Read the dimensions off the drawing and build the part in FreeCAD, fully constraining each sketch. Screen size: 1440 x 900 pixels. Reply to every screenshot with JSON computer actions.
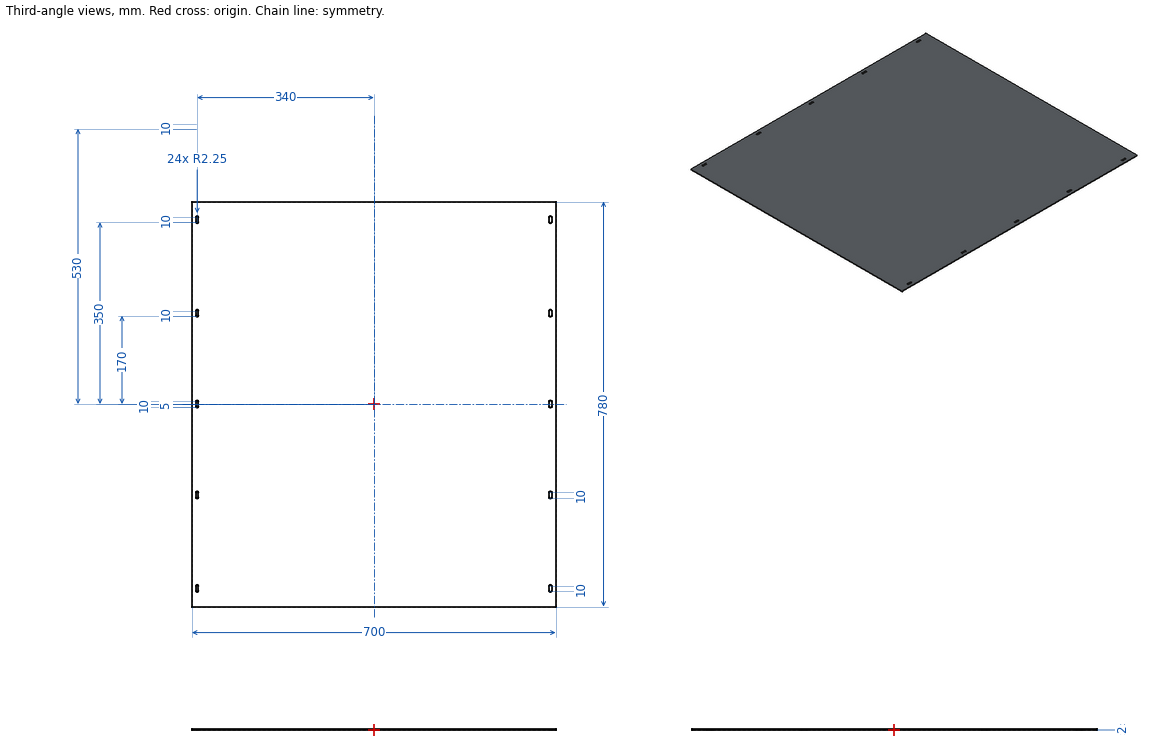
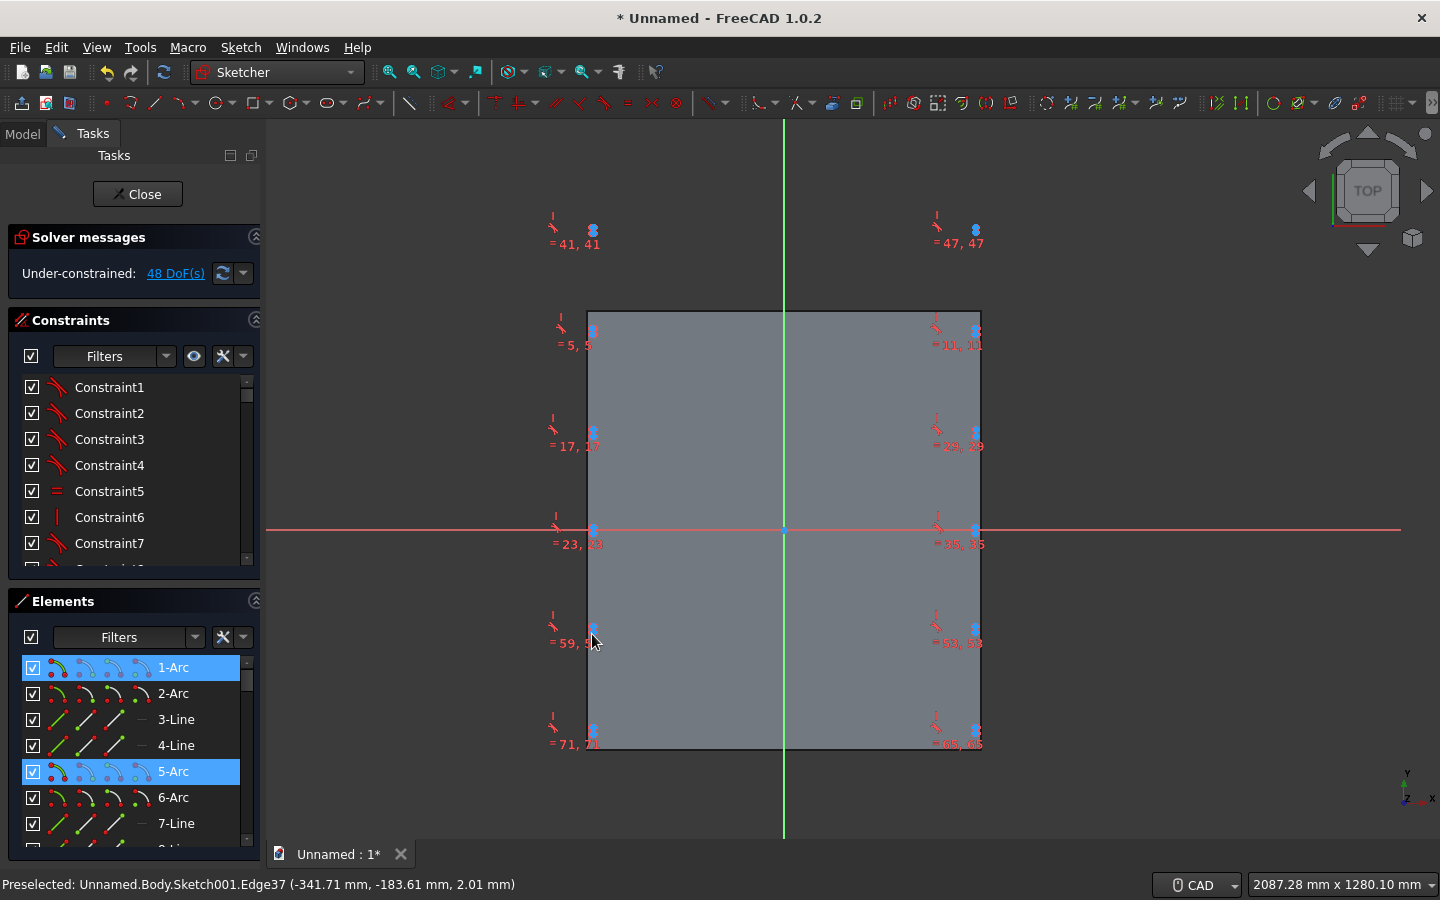
{"action": "scroll", "coordinate": [975, 735], "scroll_direction": "up", "scroll_amount": 12}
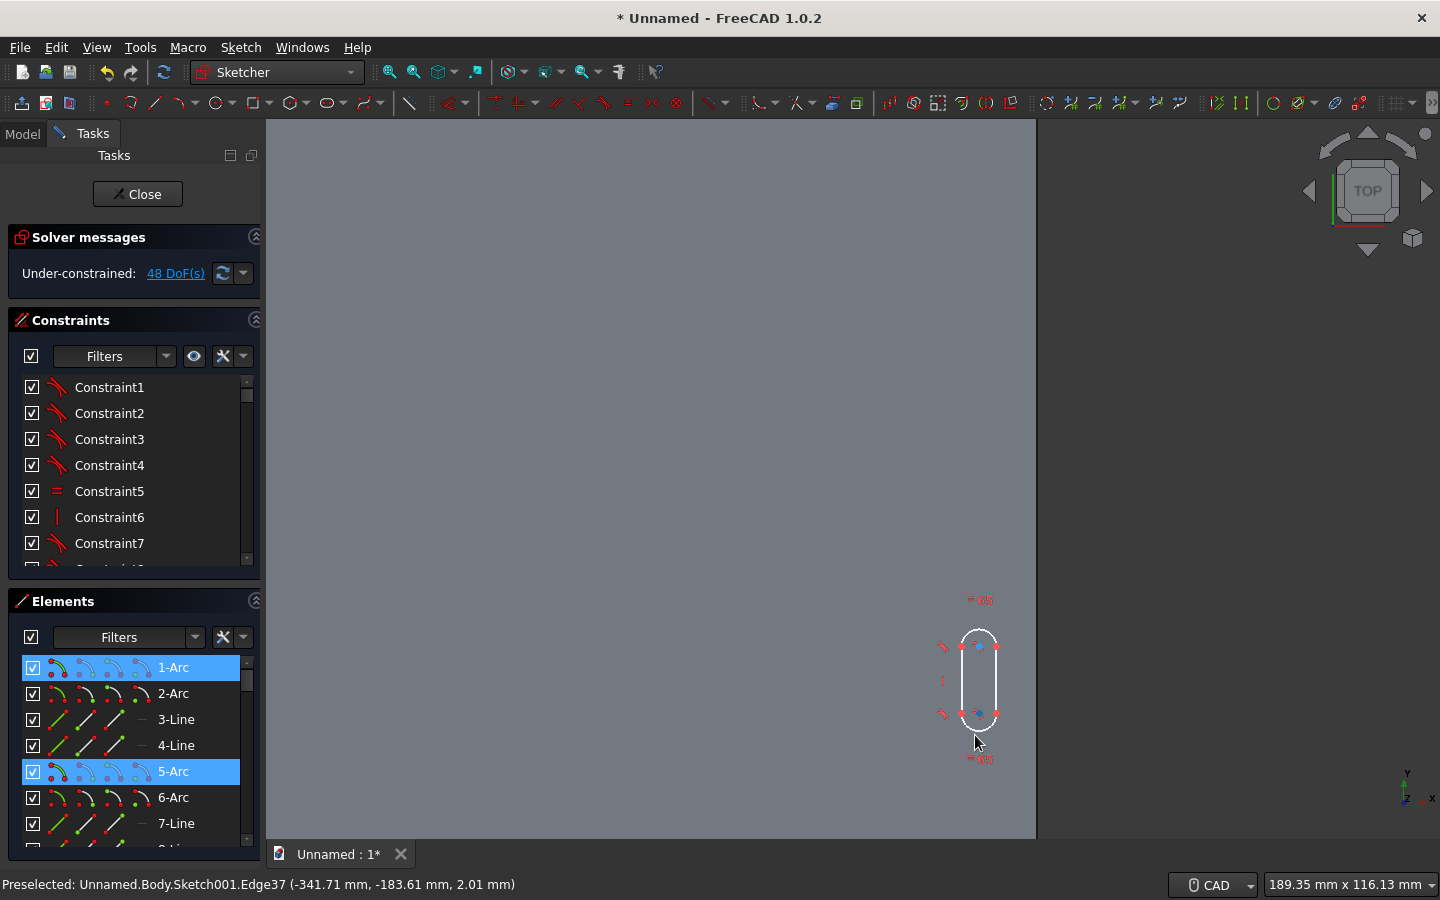
{"action": "left_click", "coordinate": [969, 728]}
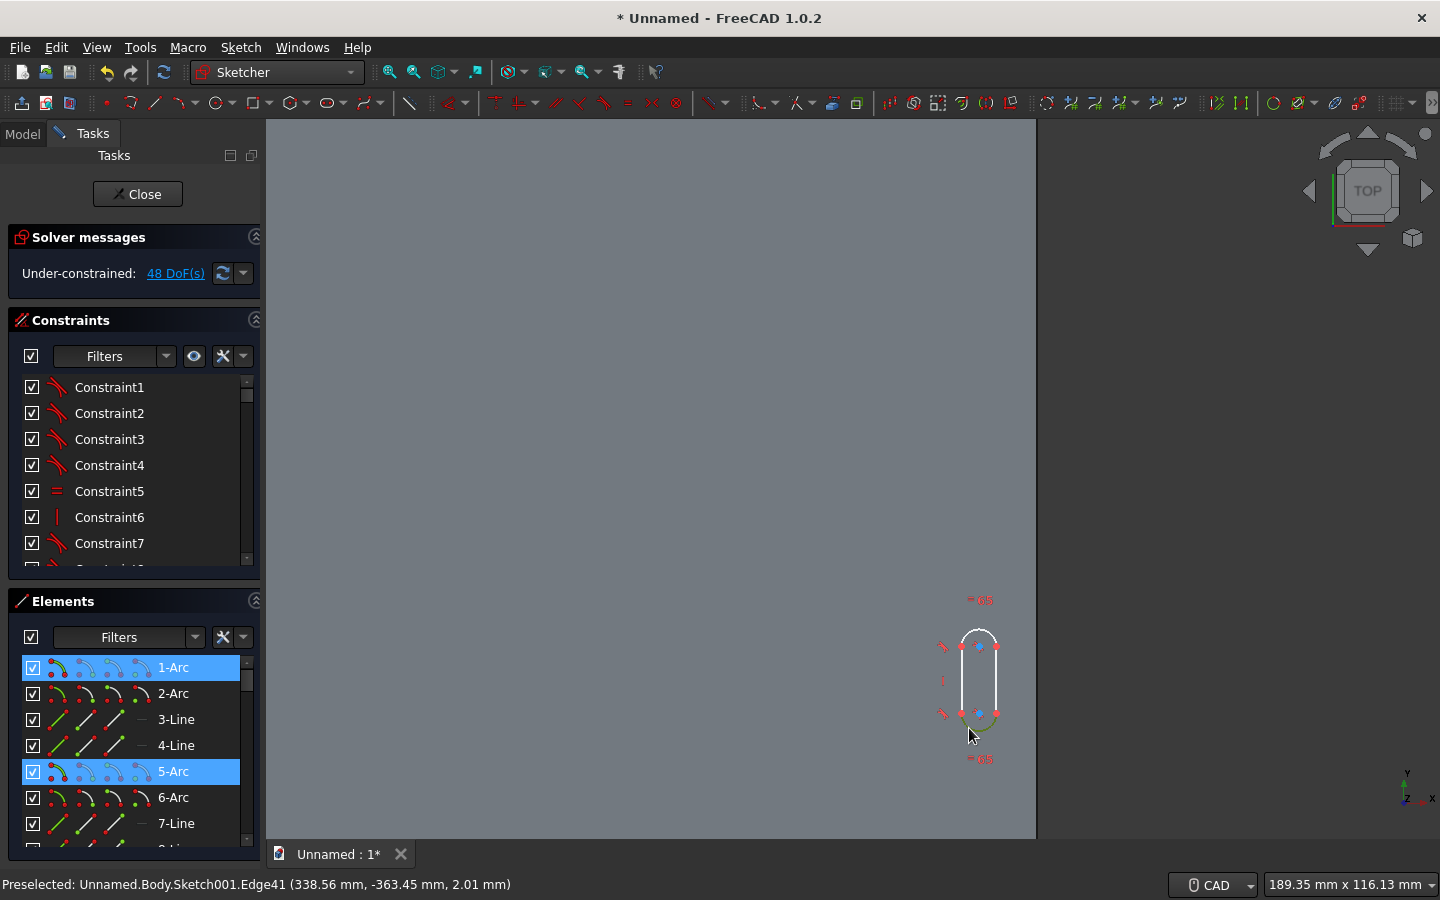
{"action": "scroll", "coordinate": [976, 735], "scroll_direction": "down", "scroll_amount": 12}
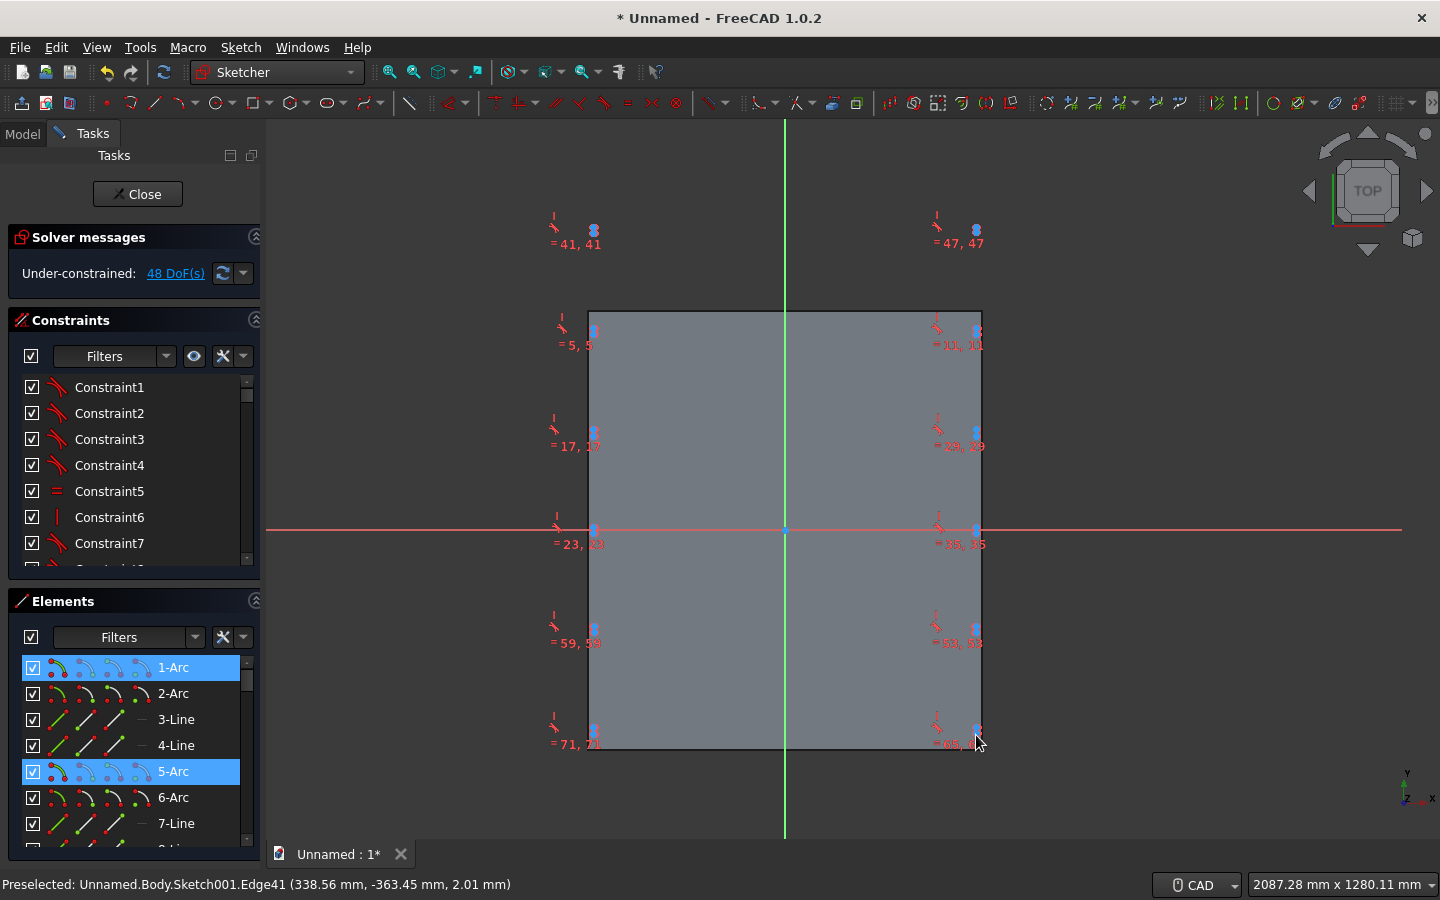
{"action": "scroll", "coordinate": [593, 735], "scroll_direction": "up", "scroll_amount": 13}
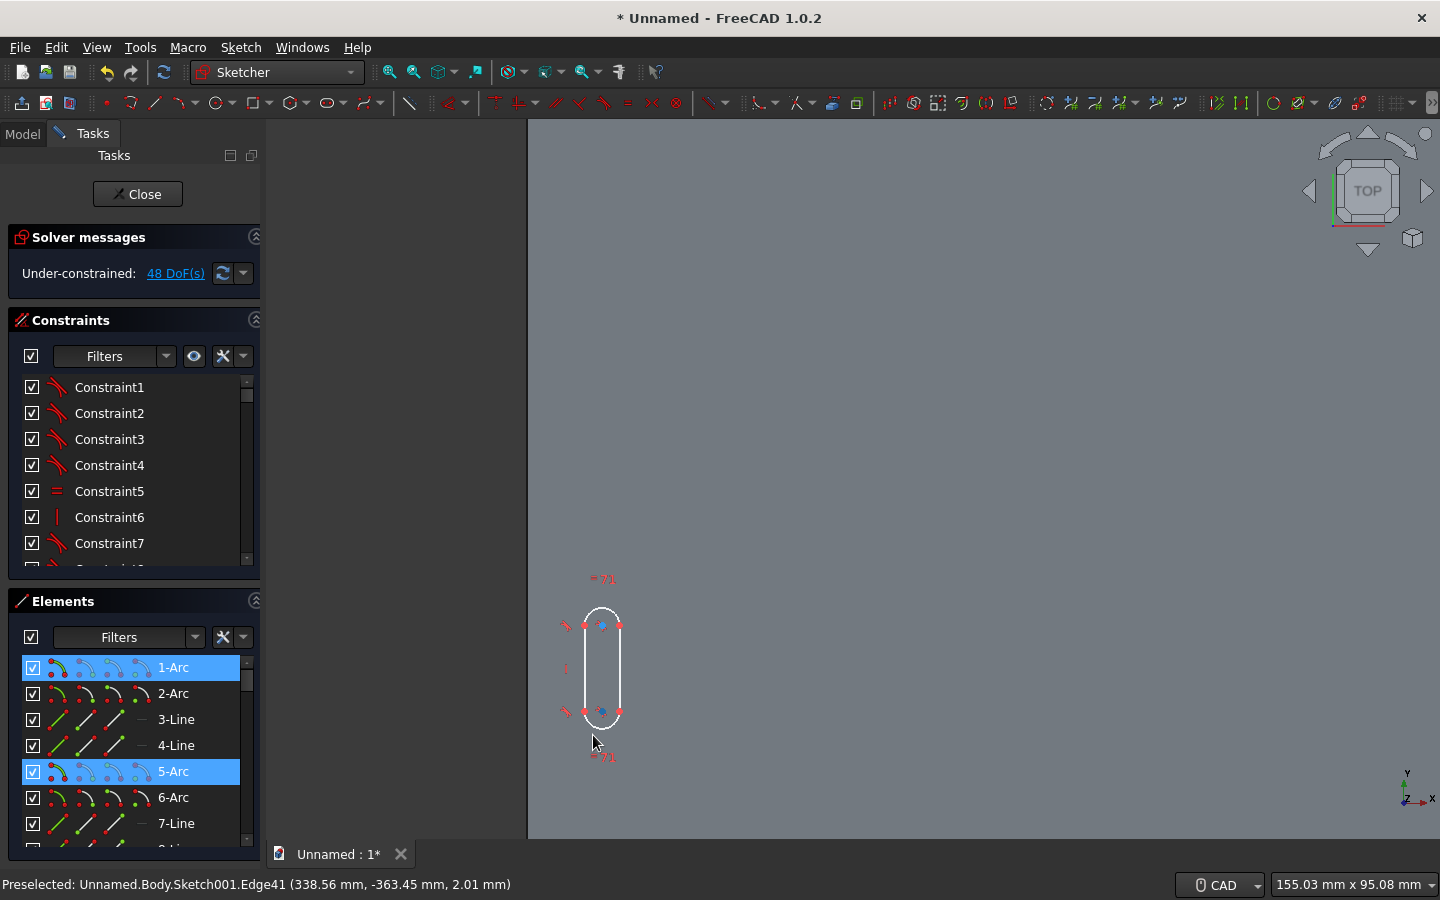
{"action": "left_click", "coordinate": [592, 725]}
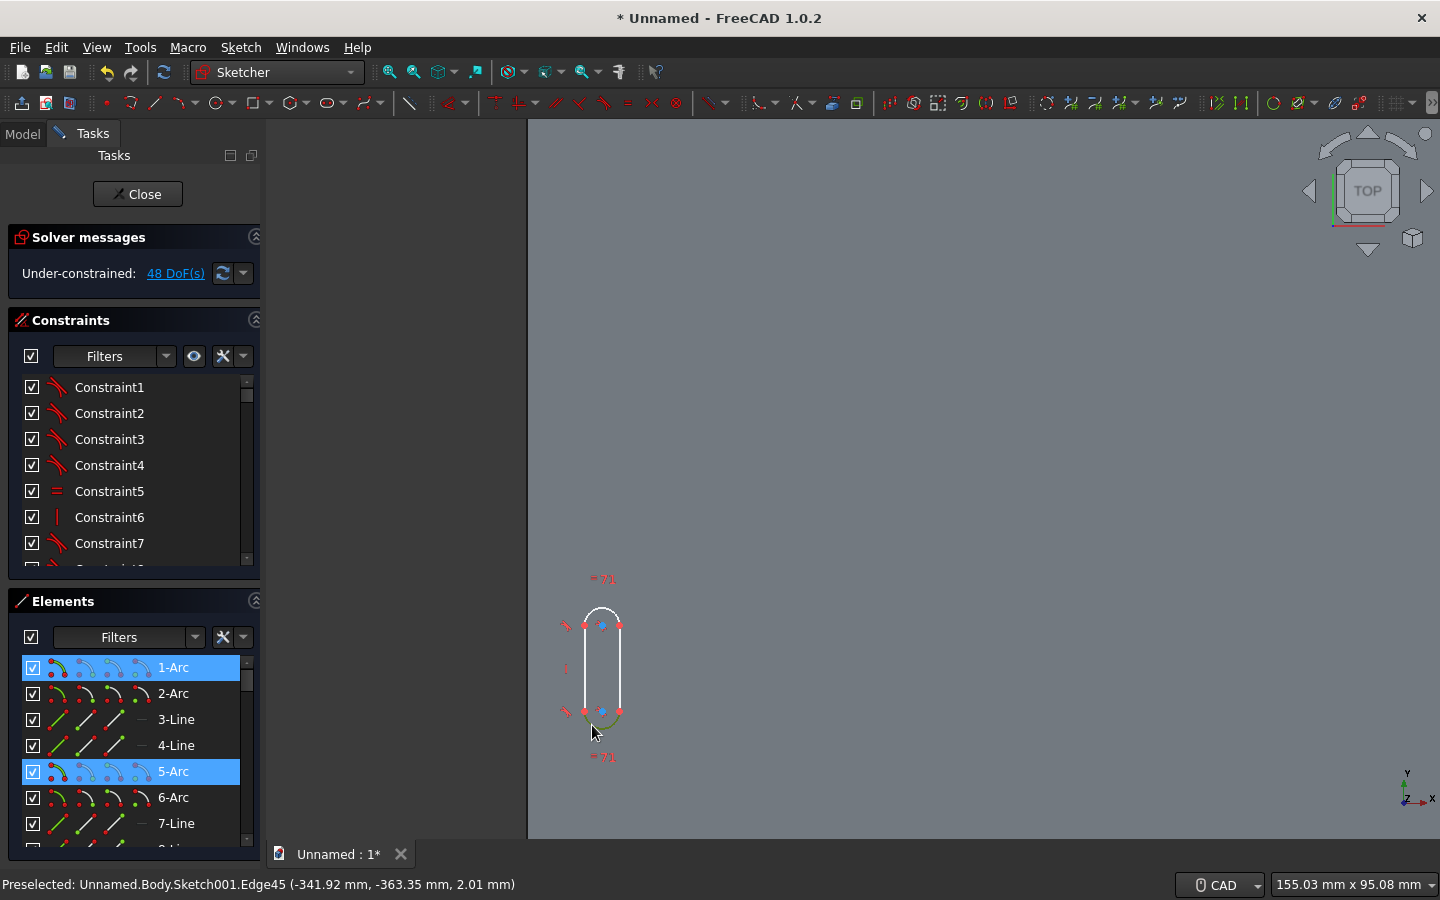
{"action": "key", "text": "e"}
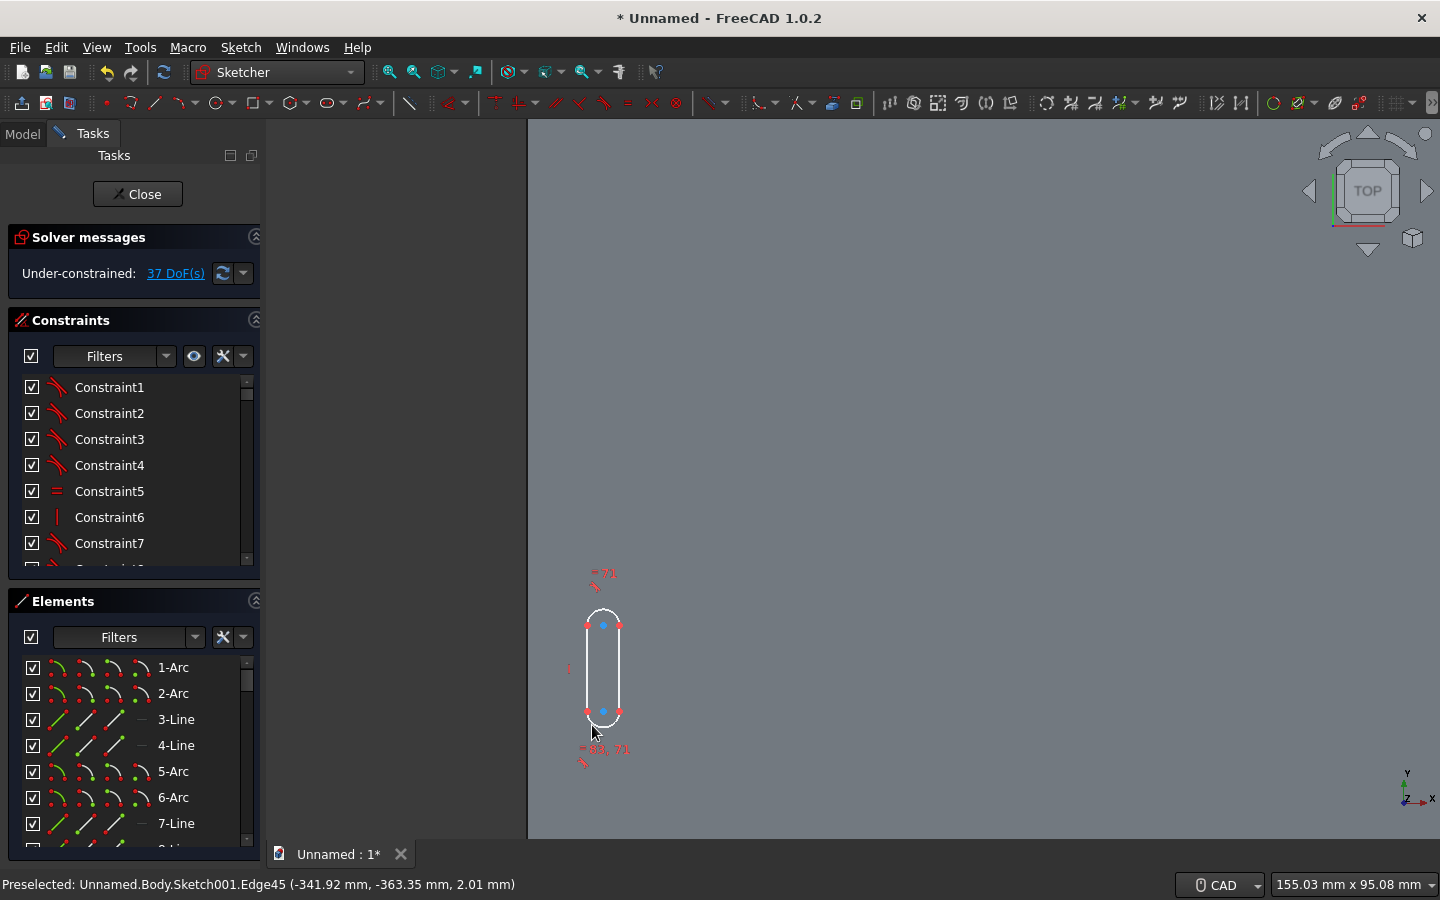
{"action": "scroll", "coordinate": [592, 735], "scroll_direction": "down", "scroll_amount": 13}